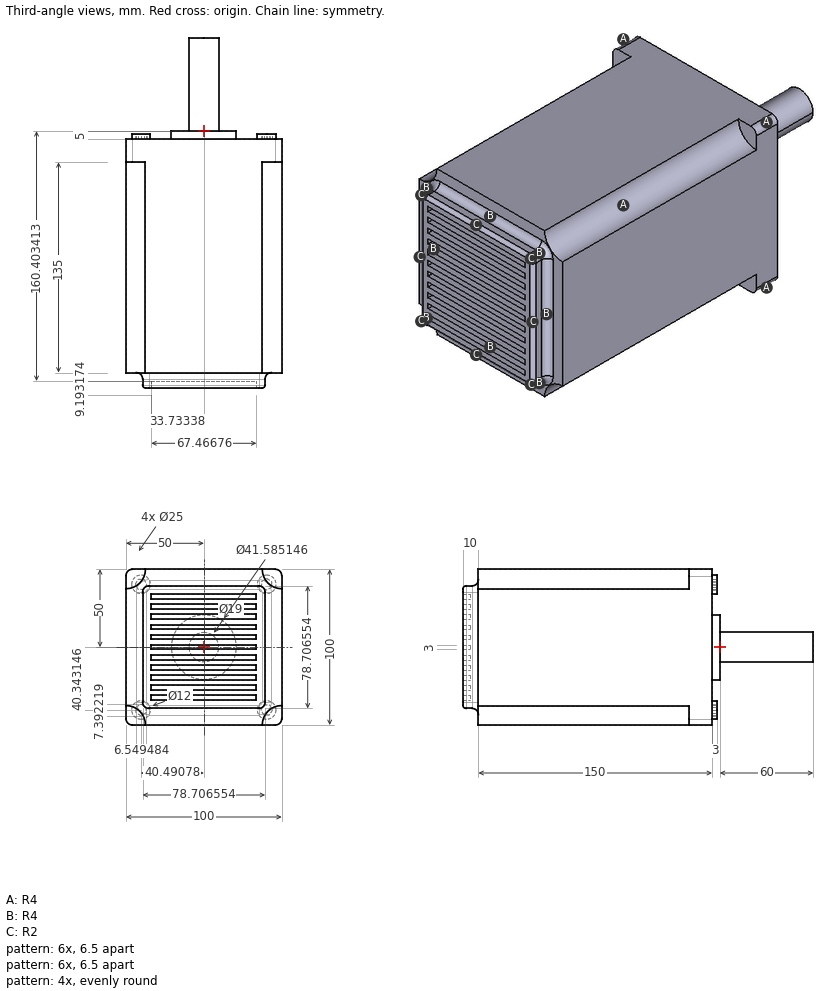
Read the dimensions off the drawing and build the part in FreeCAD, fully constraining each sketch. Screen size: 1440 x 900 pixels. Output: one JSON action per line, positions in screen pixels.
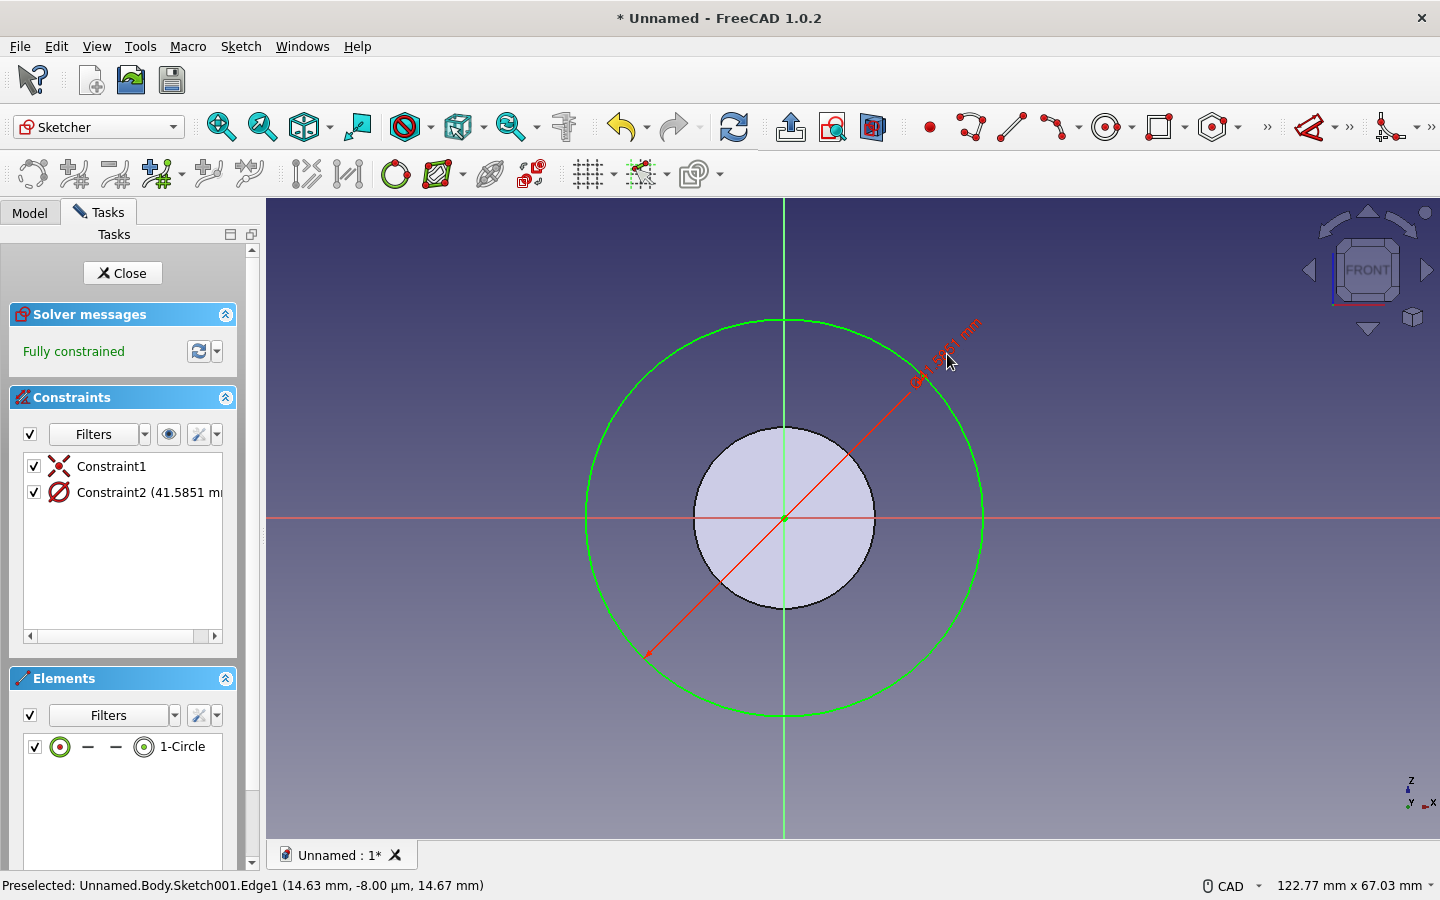
{"action": "left_click", "coordinate": [123, 273]}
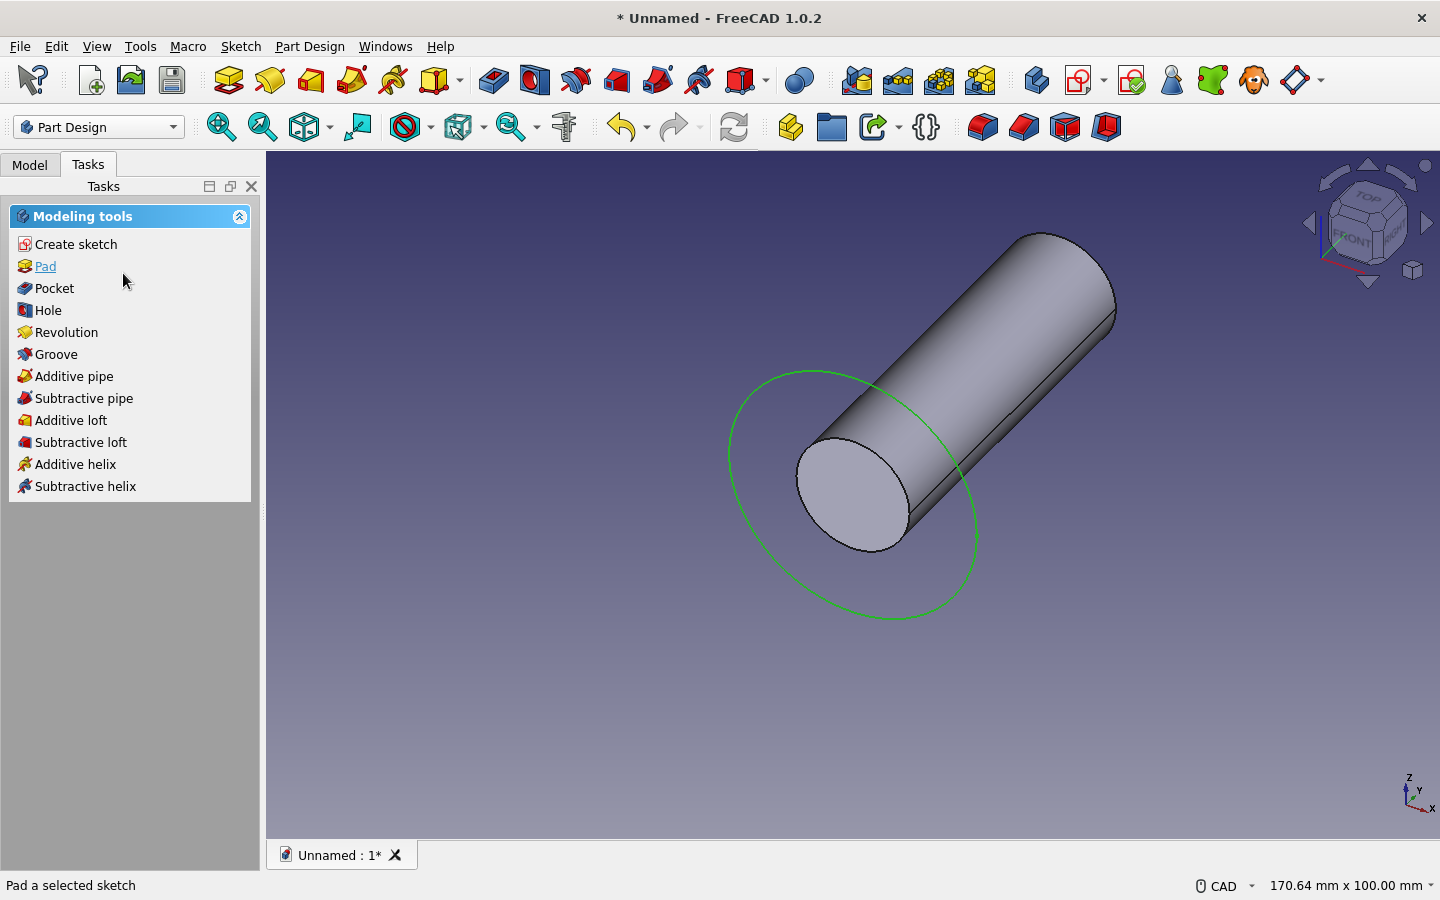
{"action": "left_click", "coordinate": [229, 80]}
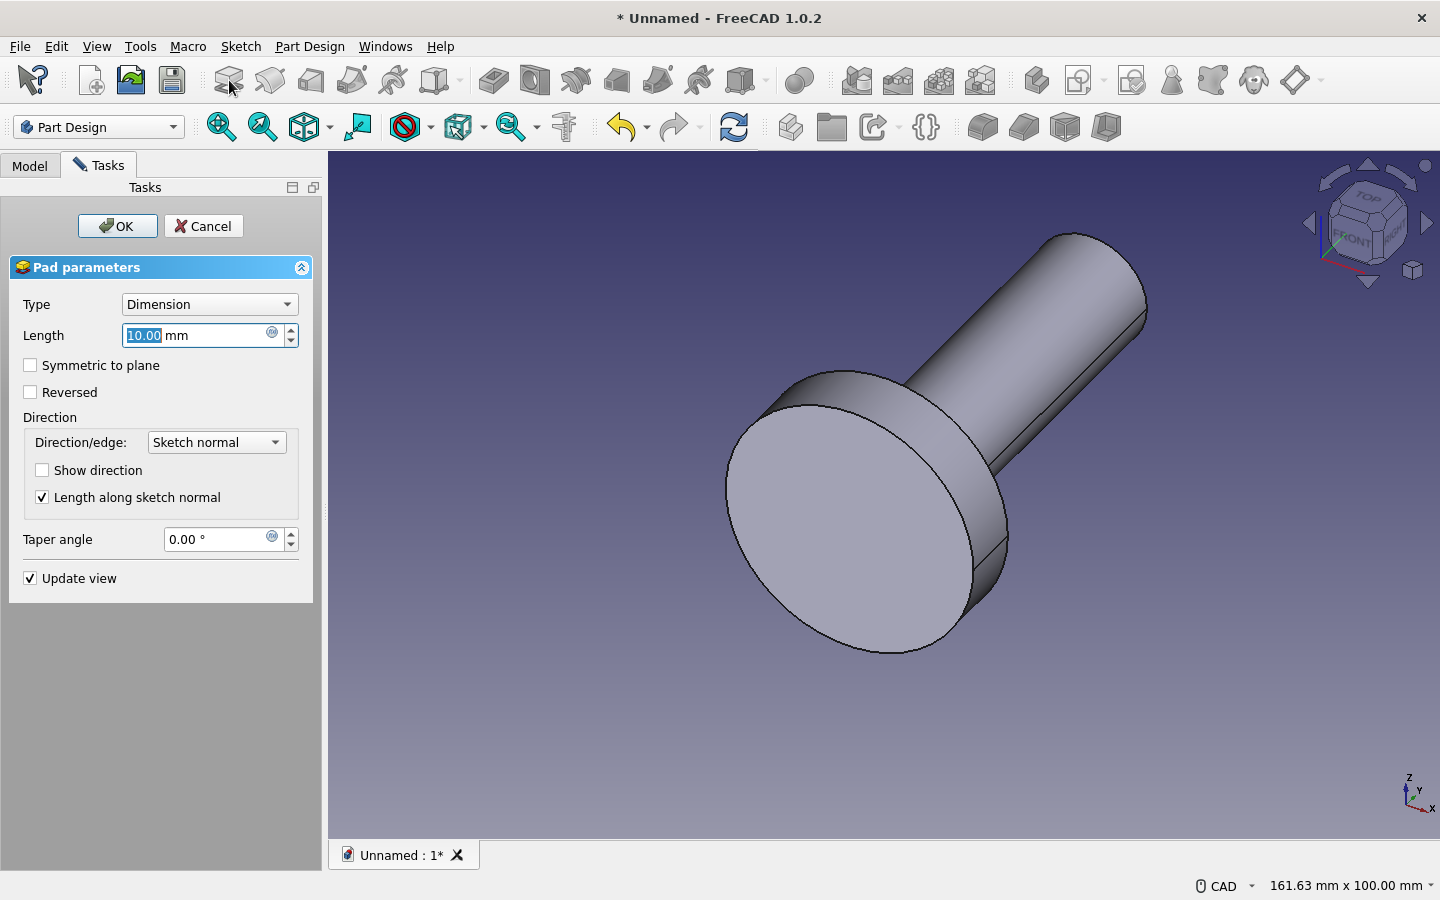
{"action": "type", "text": "5"}
{"action": "key", "text": "Tab"}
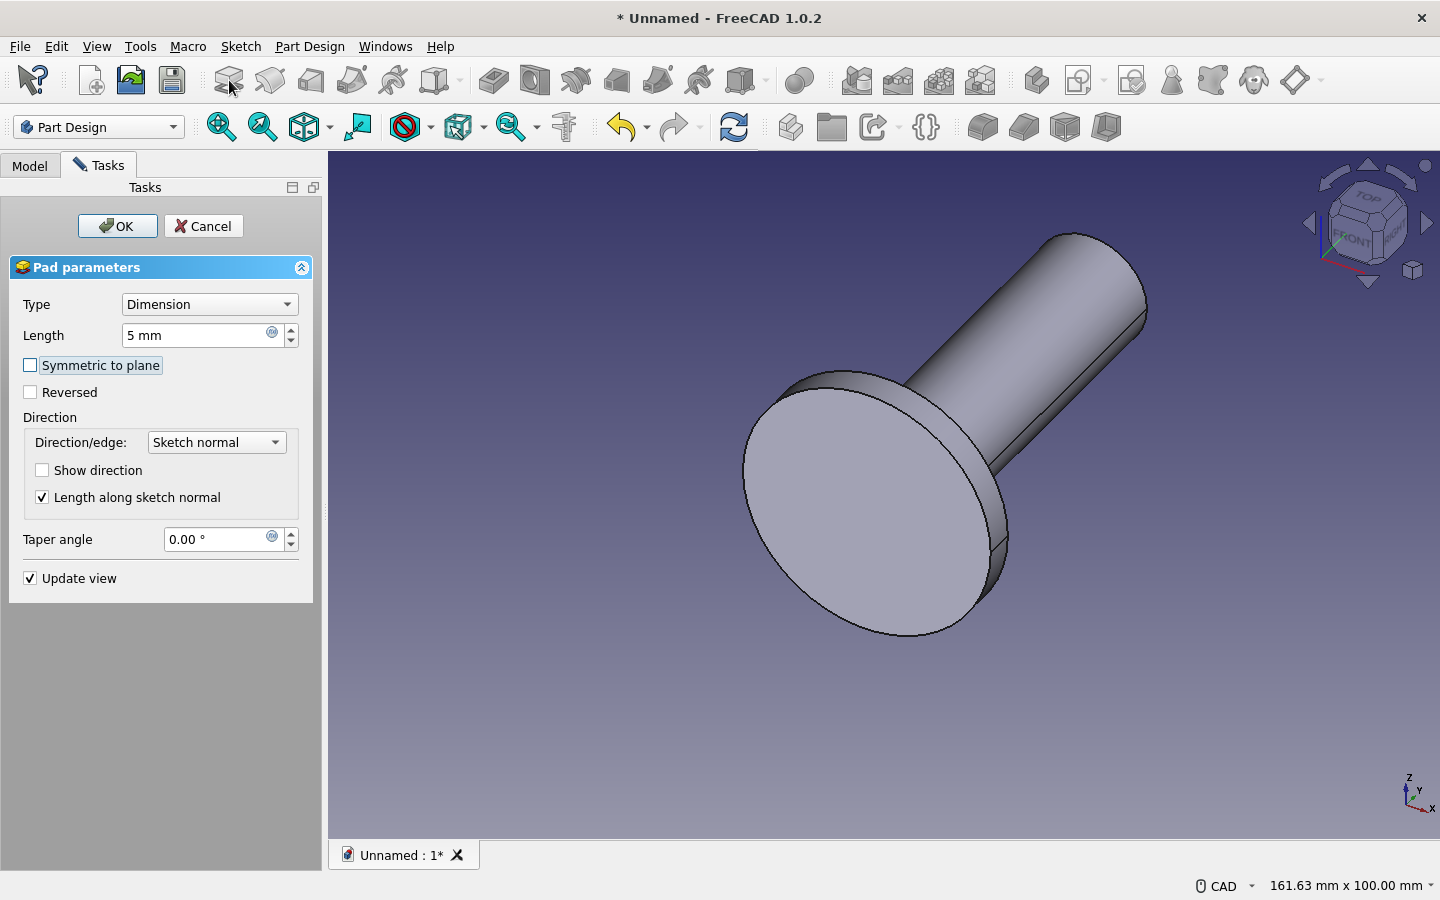
{"action": "left_click", "coordinate": [118, 226]}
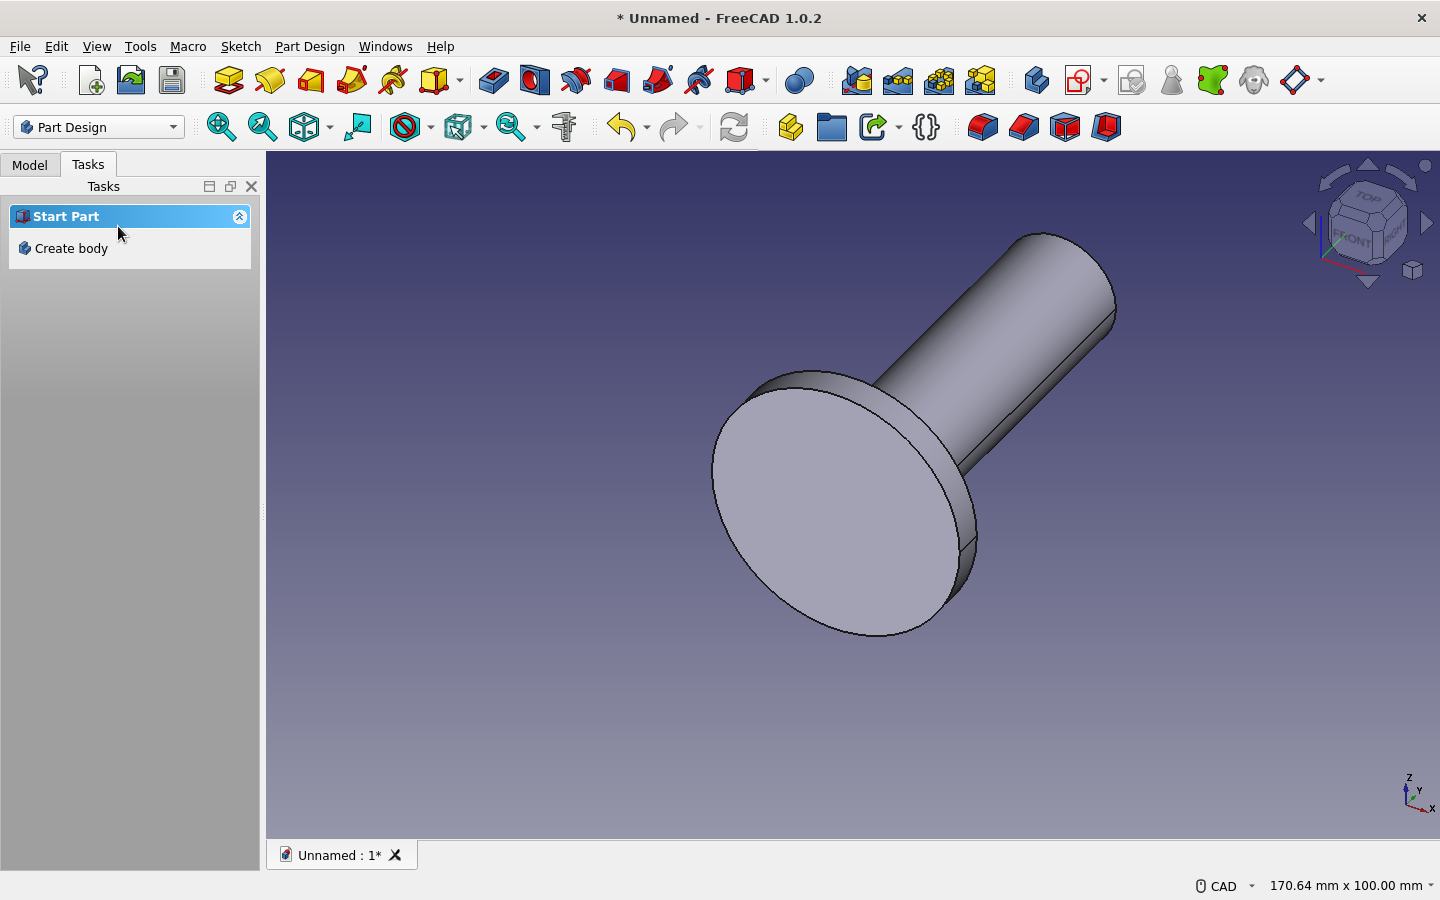
{"action": "left_click", "coordinate": [222, 128]}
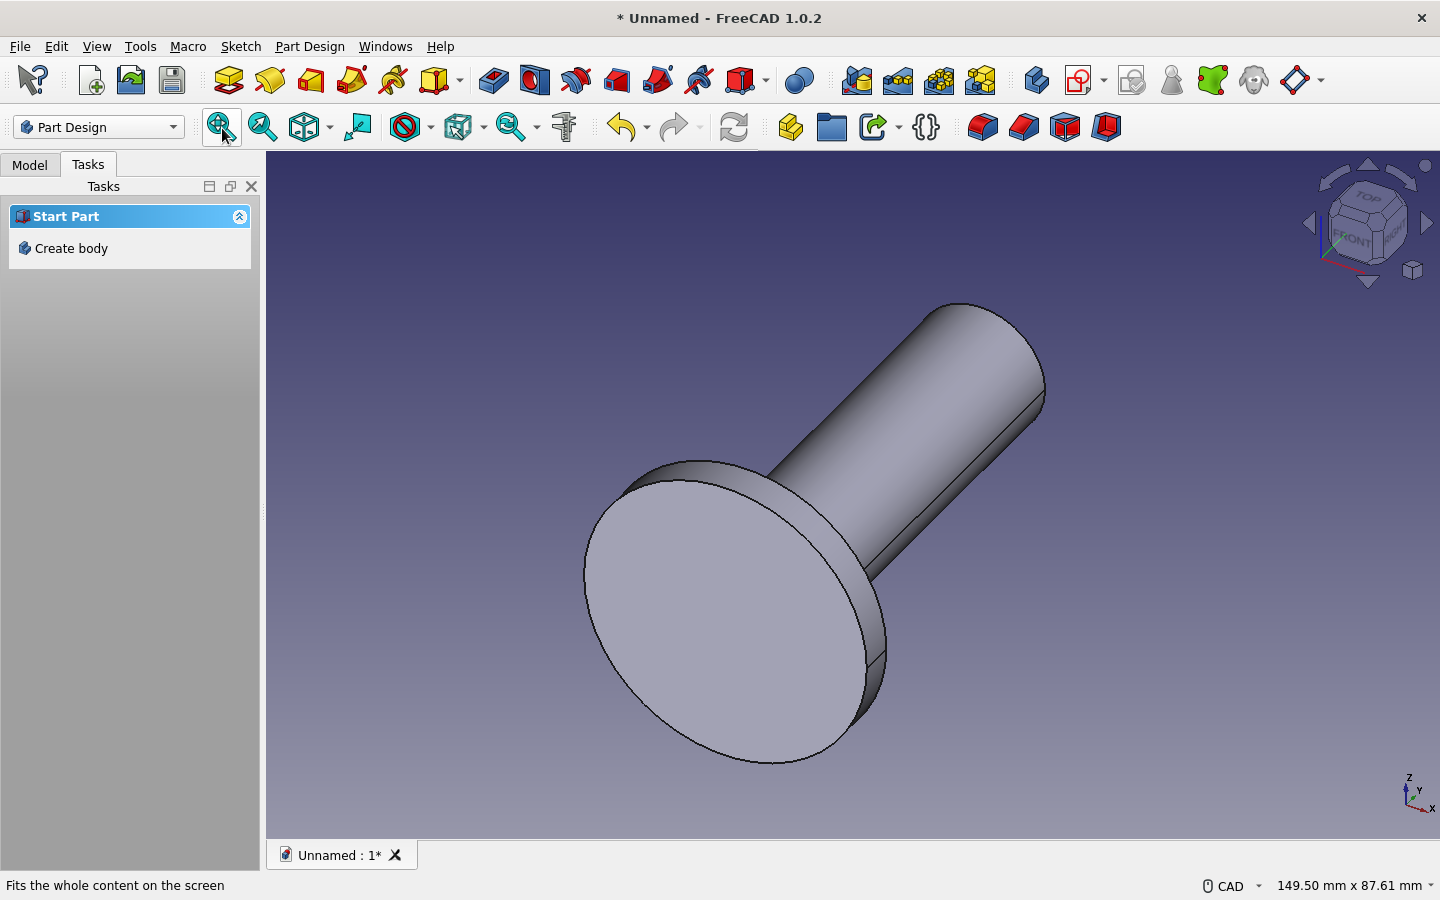
{"action": "left_click", "coordinate": [725, 621]}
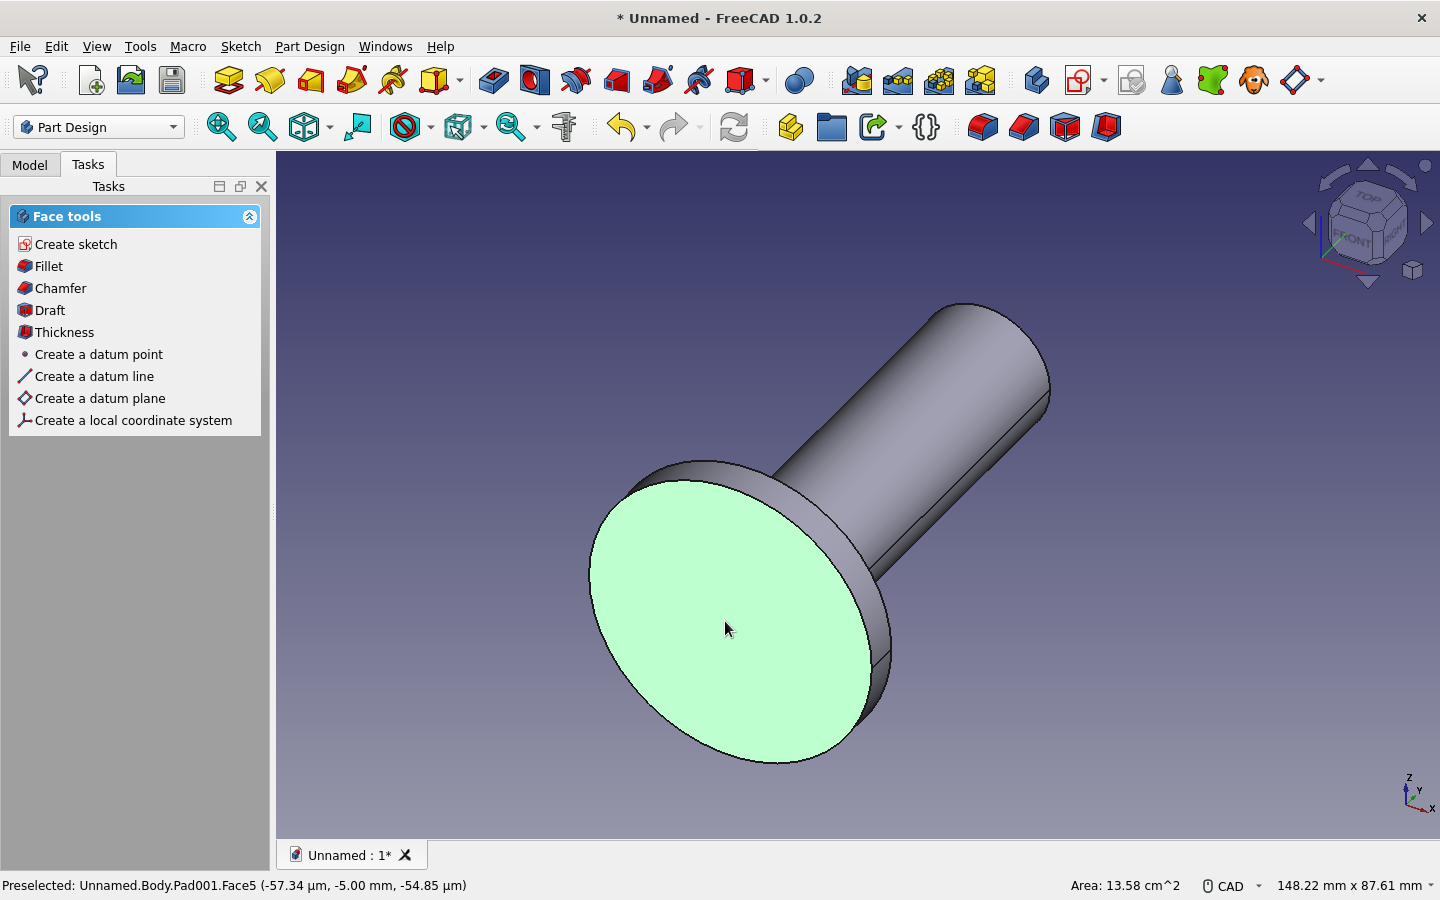
{"action": "left_click", "coordinate": [1078, 80]}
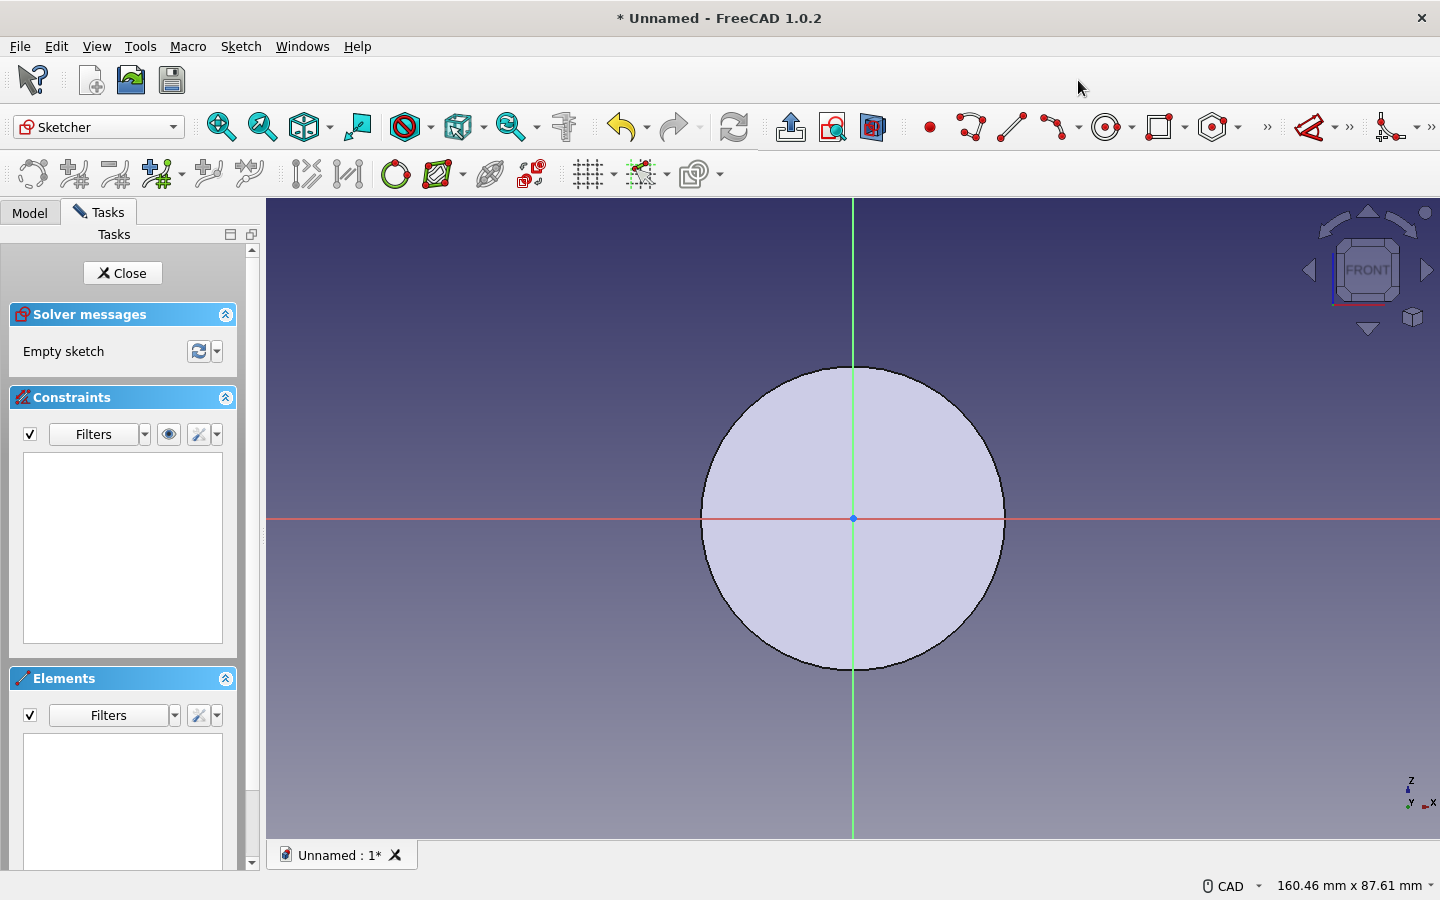
{"action": "scroll", "coordinate": [701, 518], "scroll_direction": "down", "scroll_amount": 3}